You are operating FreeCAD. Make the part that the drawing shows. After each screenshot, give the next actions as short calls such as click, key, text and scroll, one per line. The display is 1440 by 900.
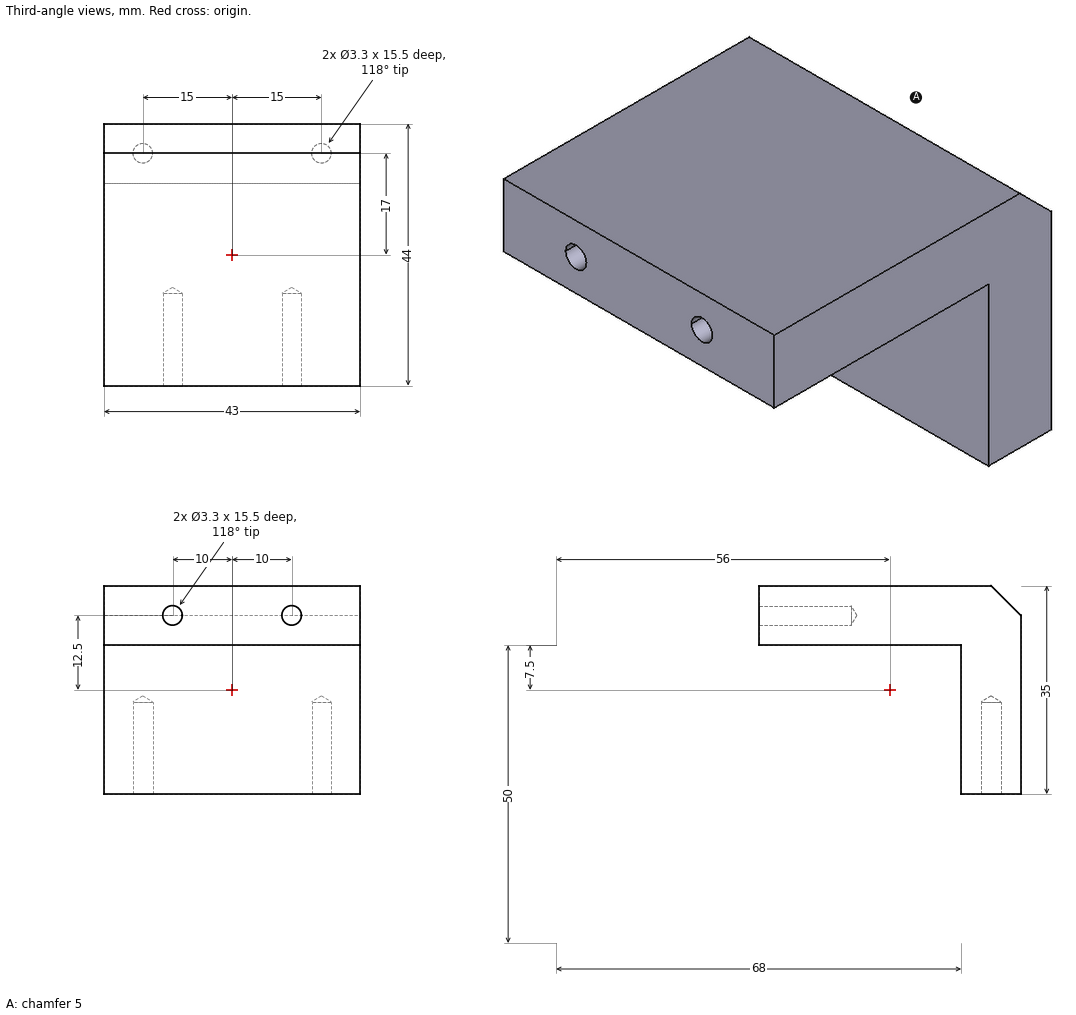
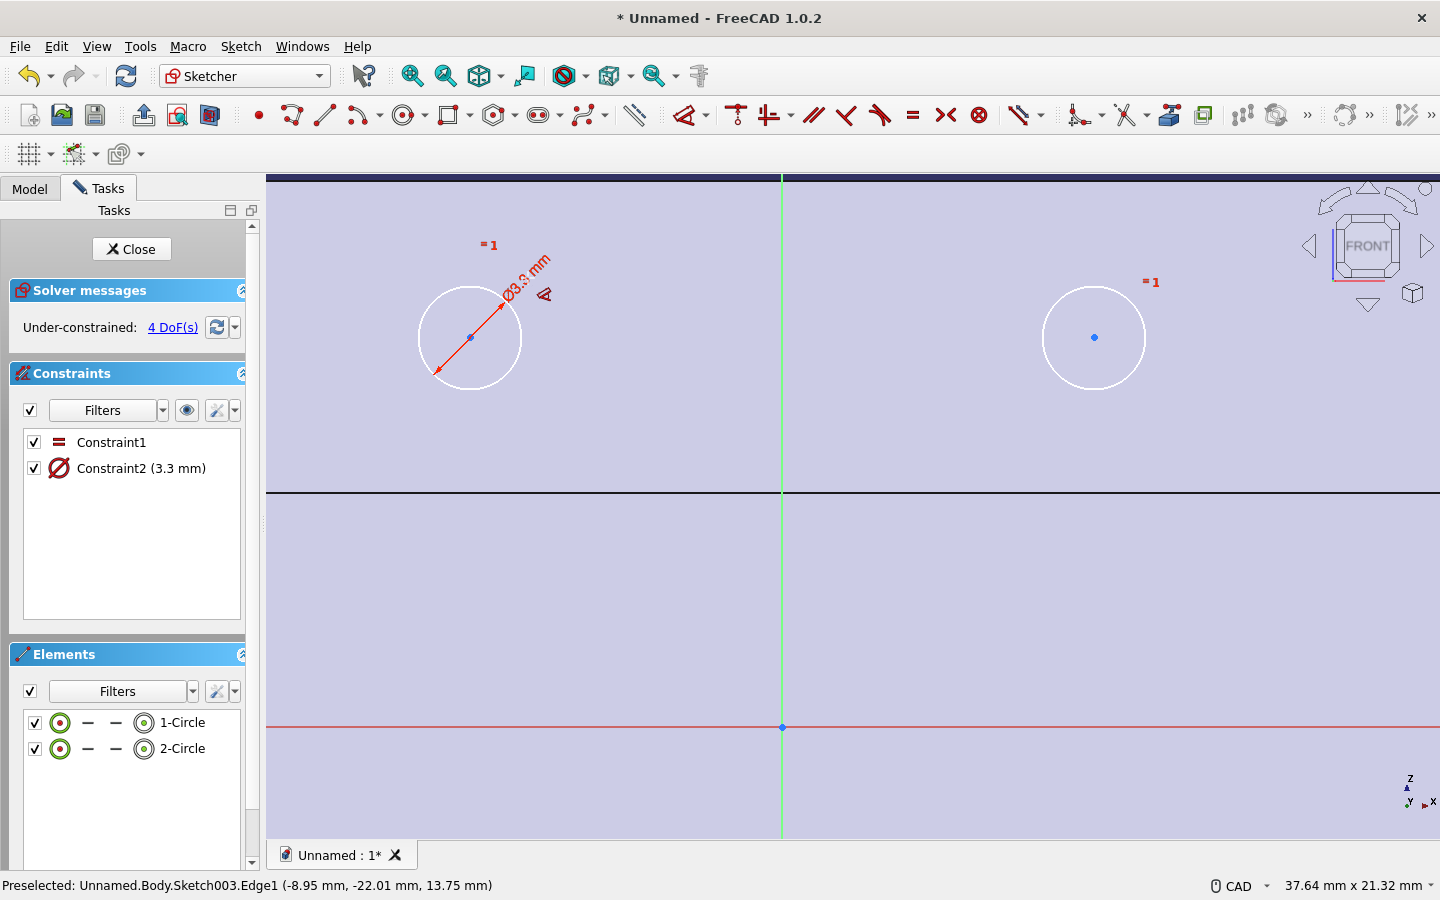
click(470, 338)
click(626, 761)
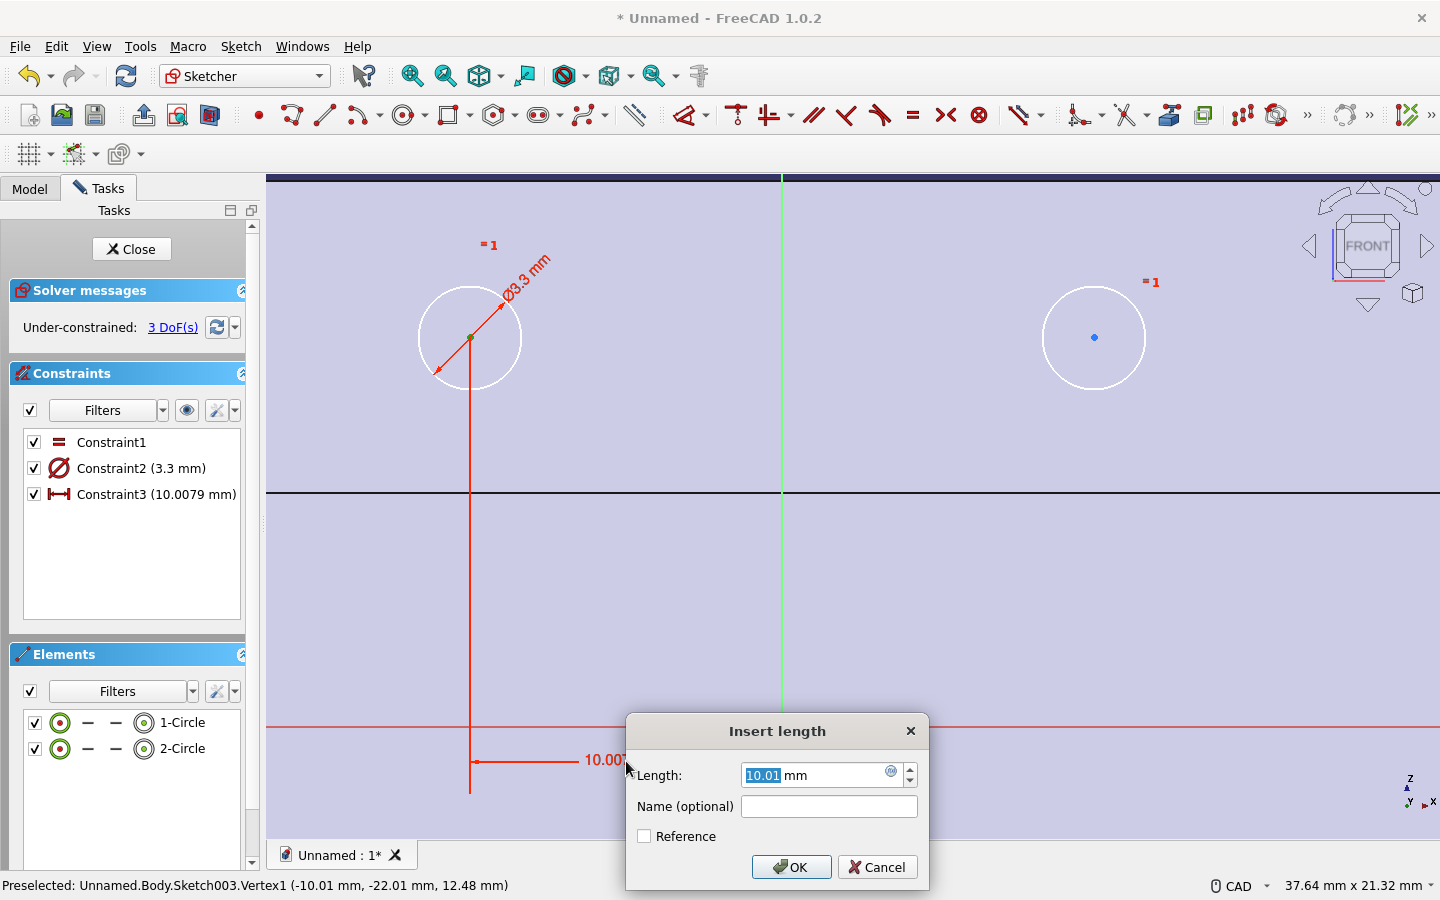
text(10)
key(Return)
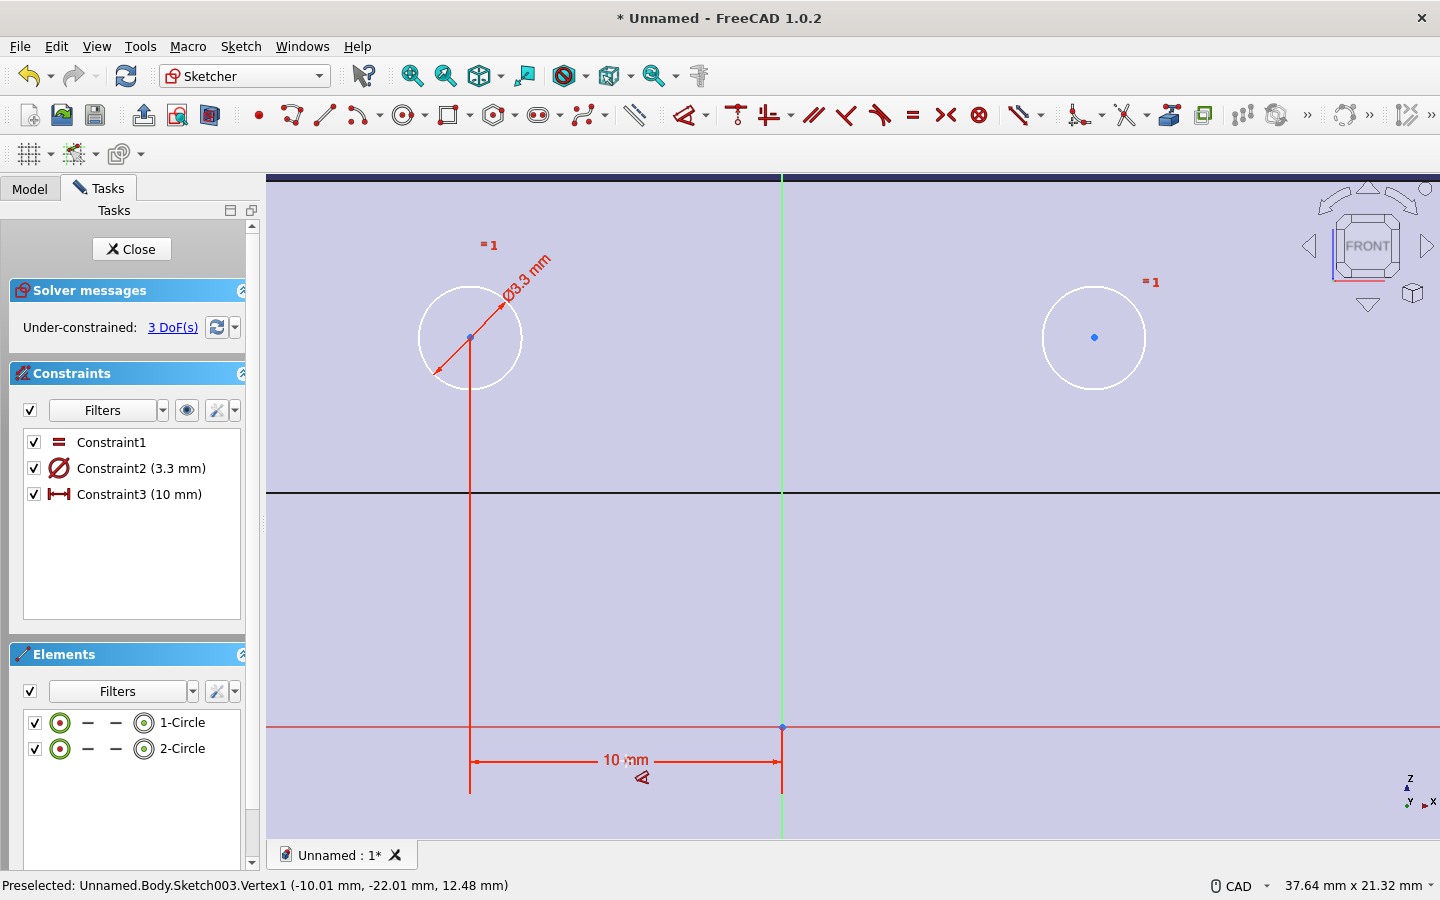
click(1094, 338)
click(938, 761)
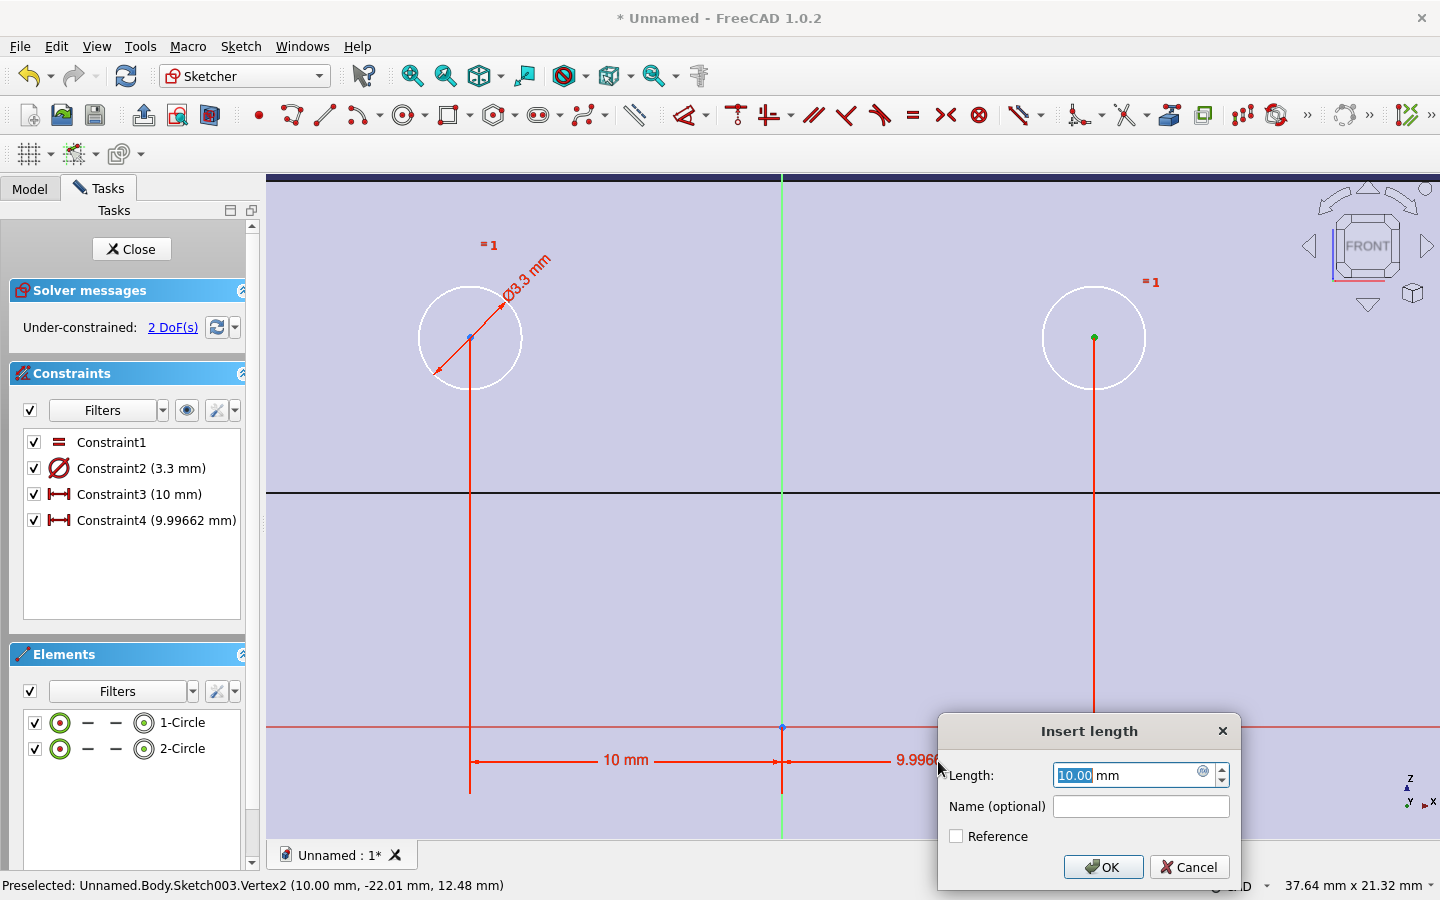
text(10)
key(Return)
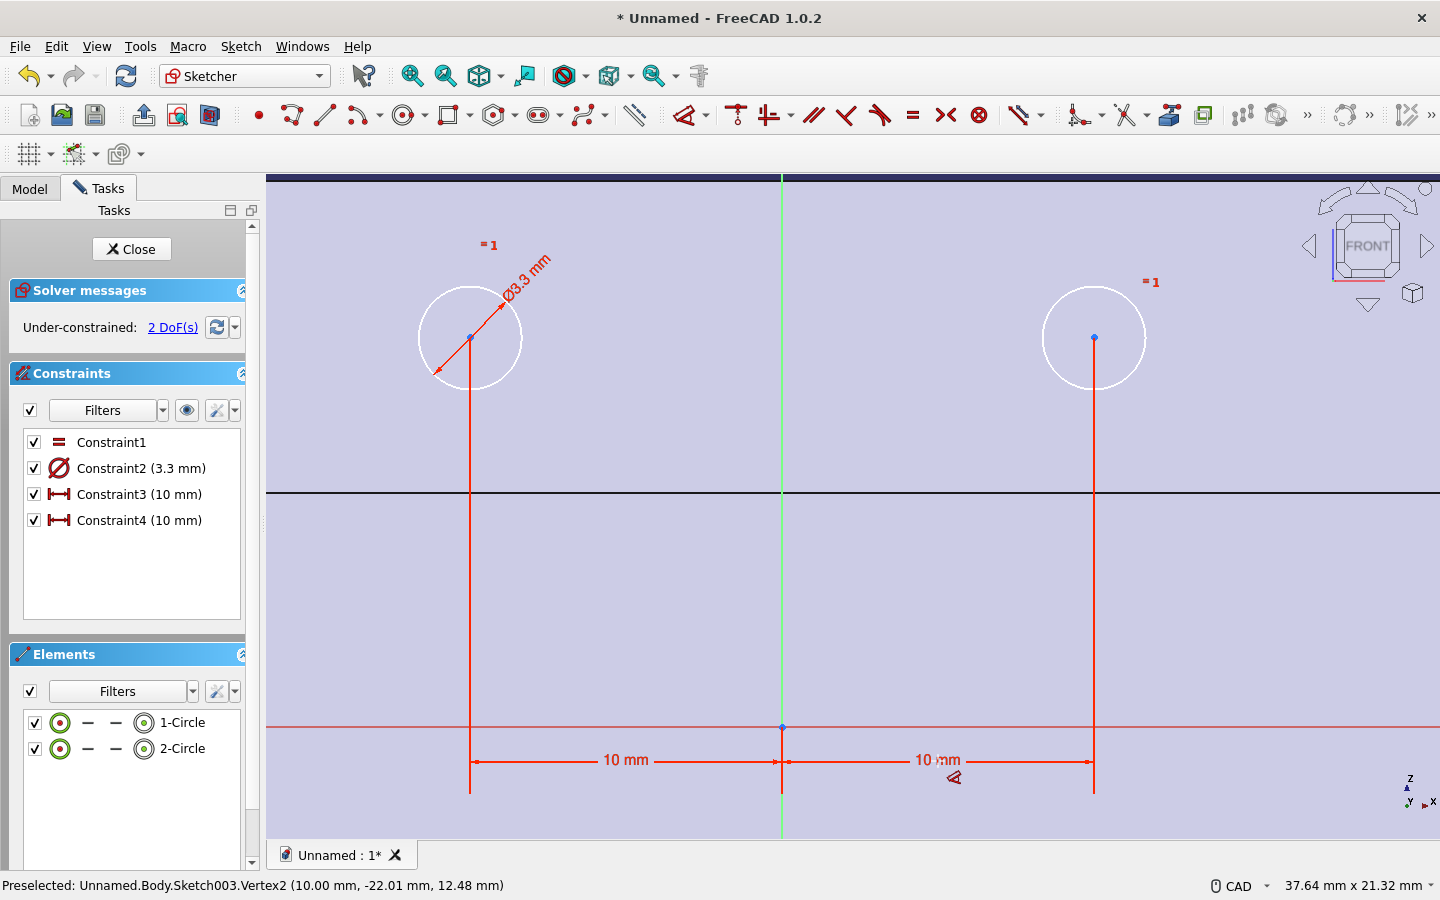
click(470, 338)
click(436, 533)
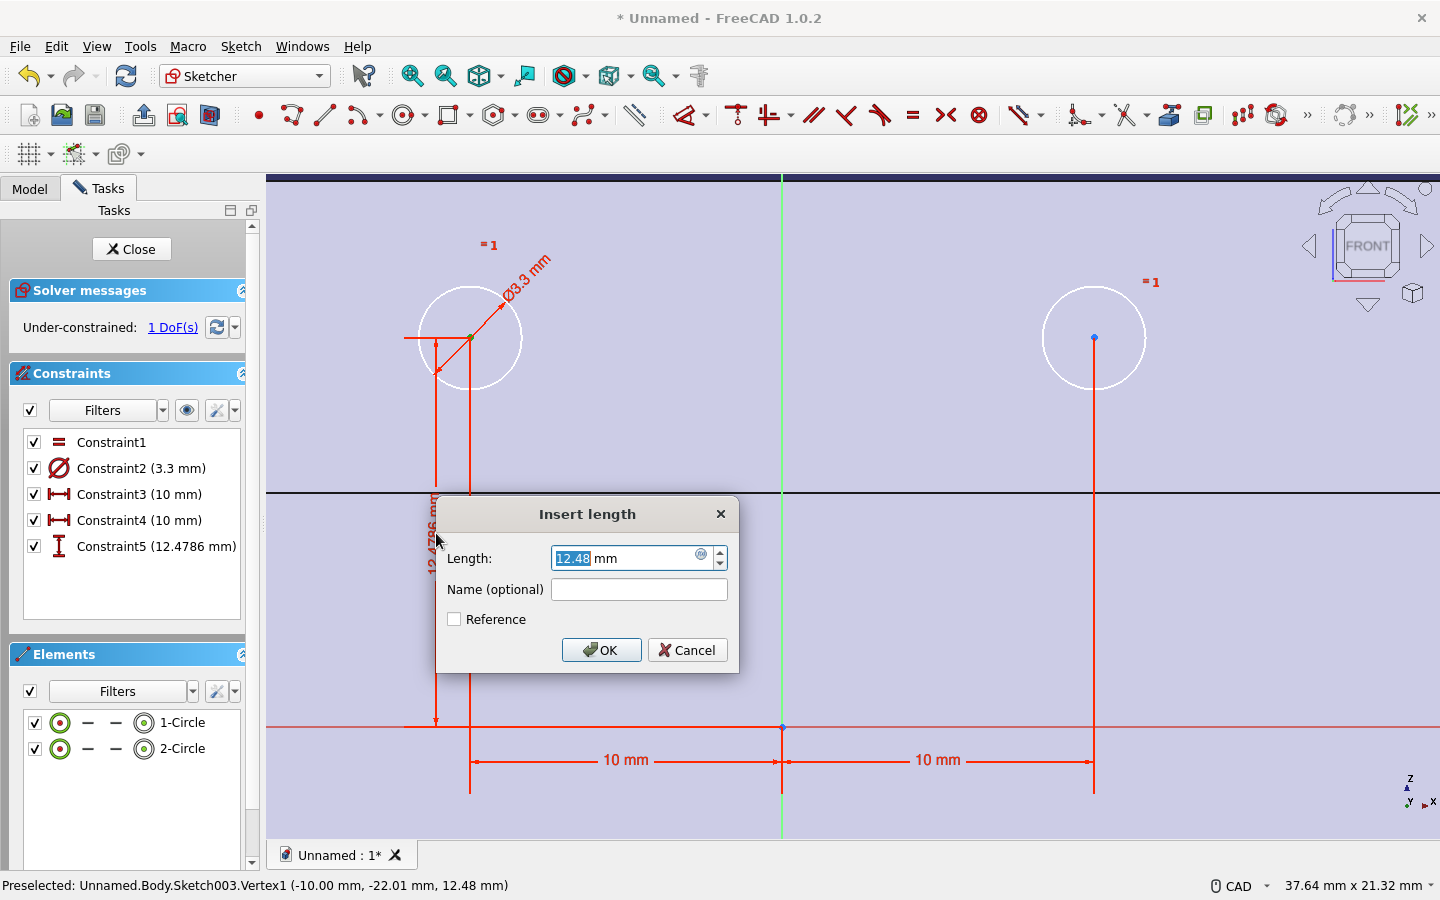
text(12.5)
key(Return)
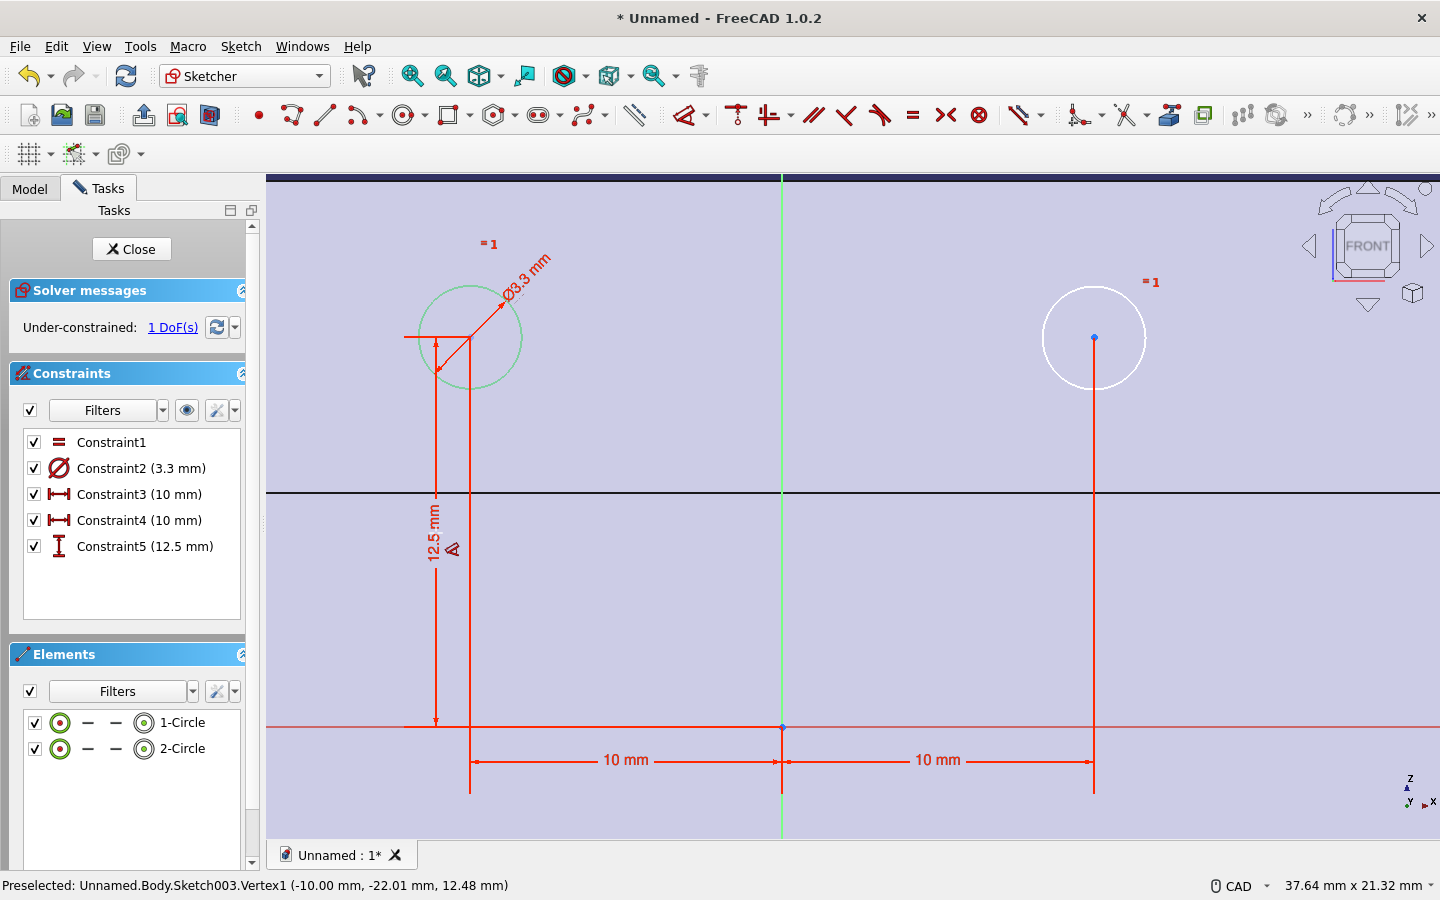
click(1094, 338)
click(1128, 533)